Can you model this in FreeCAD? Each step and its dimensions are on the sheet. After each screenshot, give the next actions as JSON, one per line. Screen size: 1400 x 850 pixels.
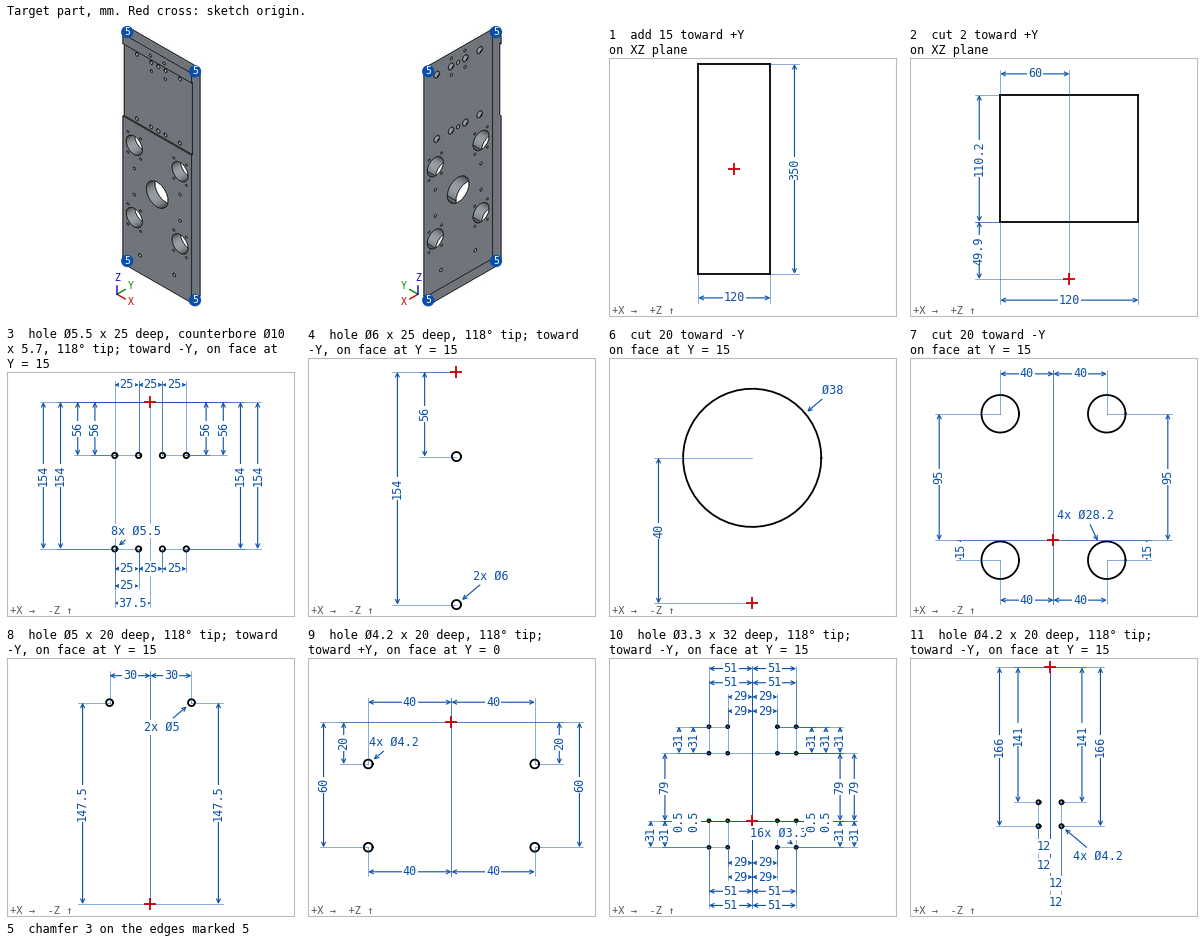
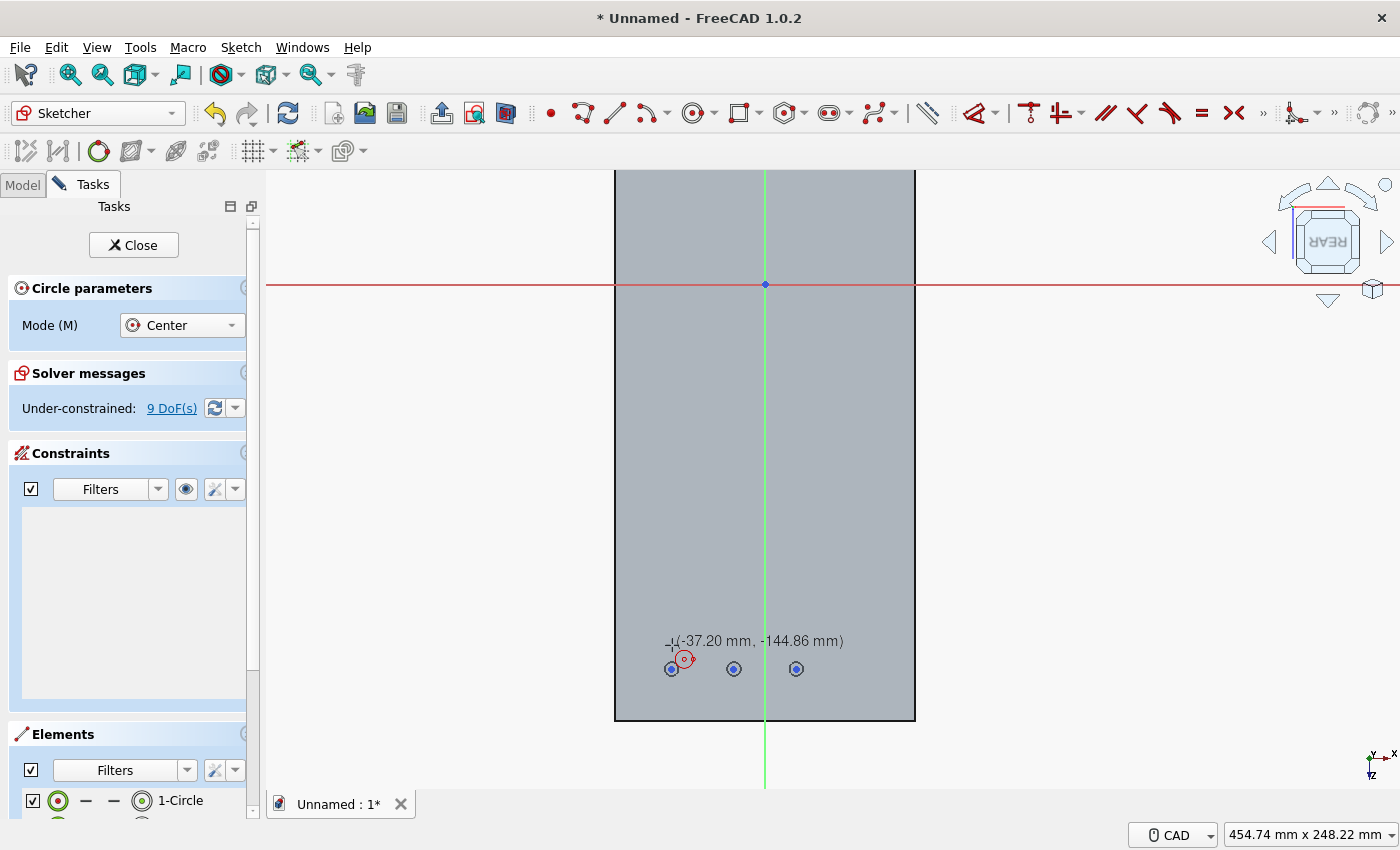
{"action": "scroll", "coordinate": [859, 669], "scroll_direction": "up", "scroll_amount": 6}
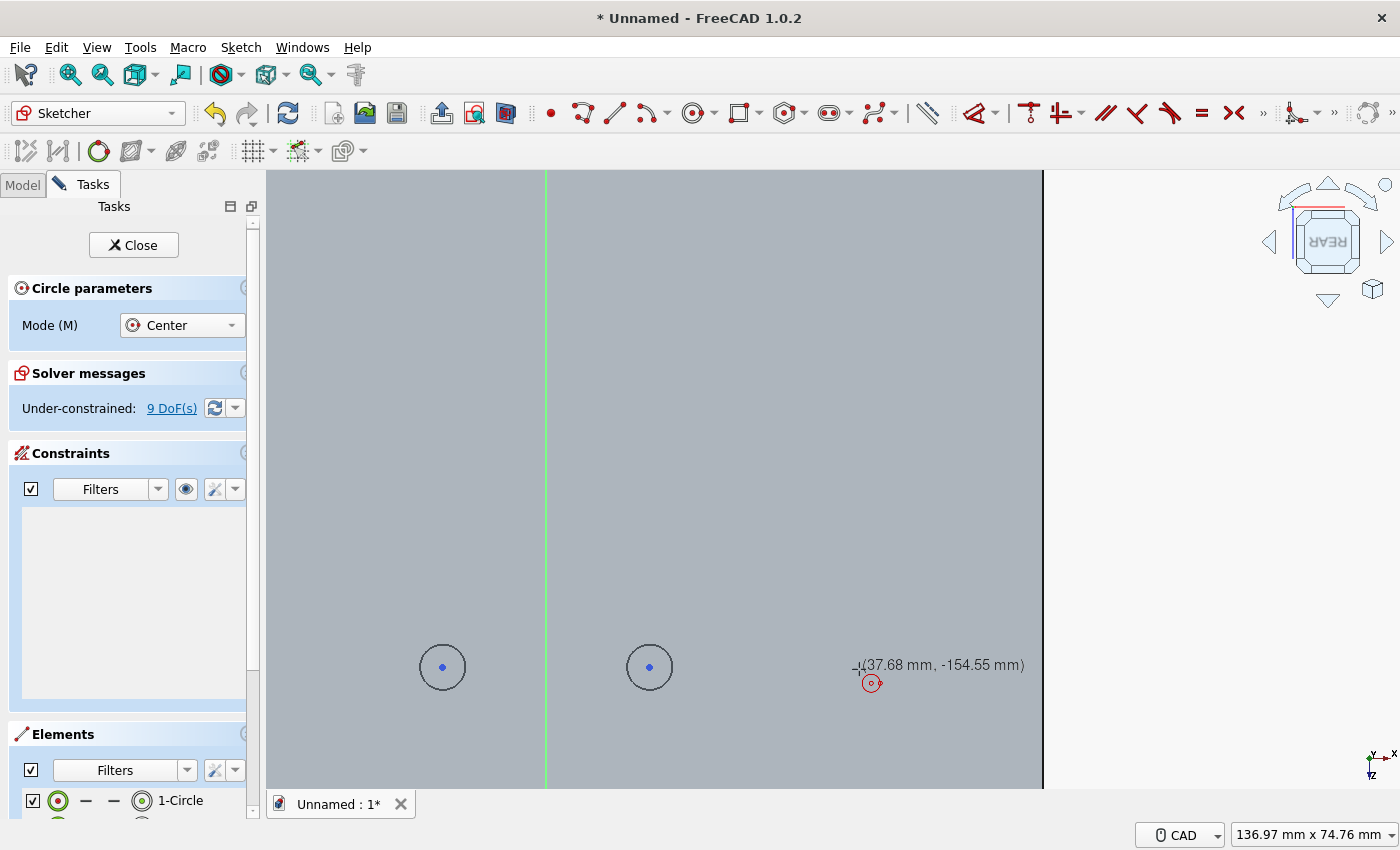
{"action": "left_click", "coordinate": [856, 666]}
{"action": "left_click", "coordinate": [872, 650]}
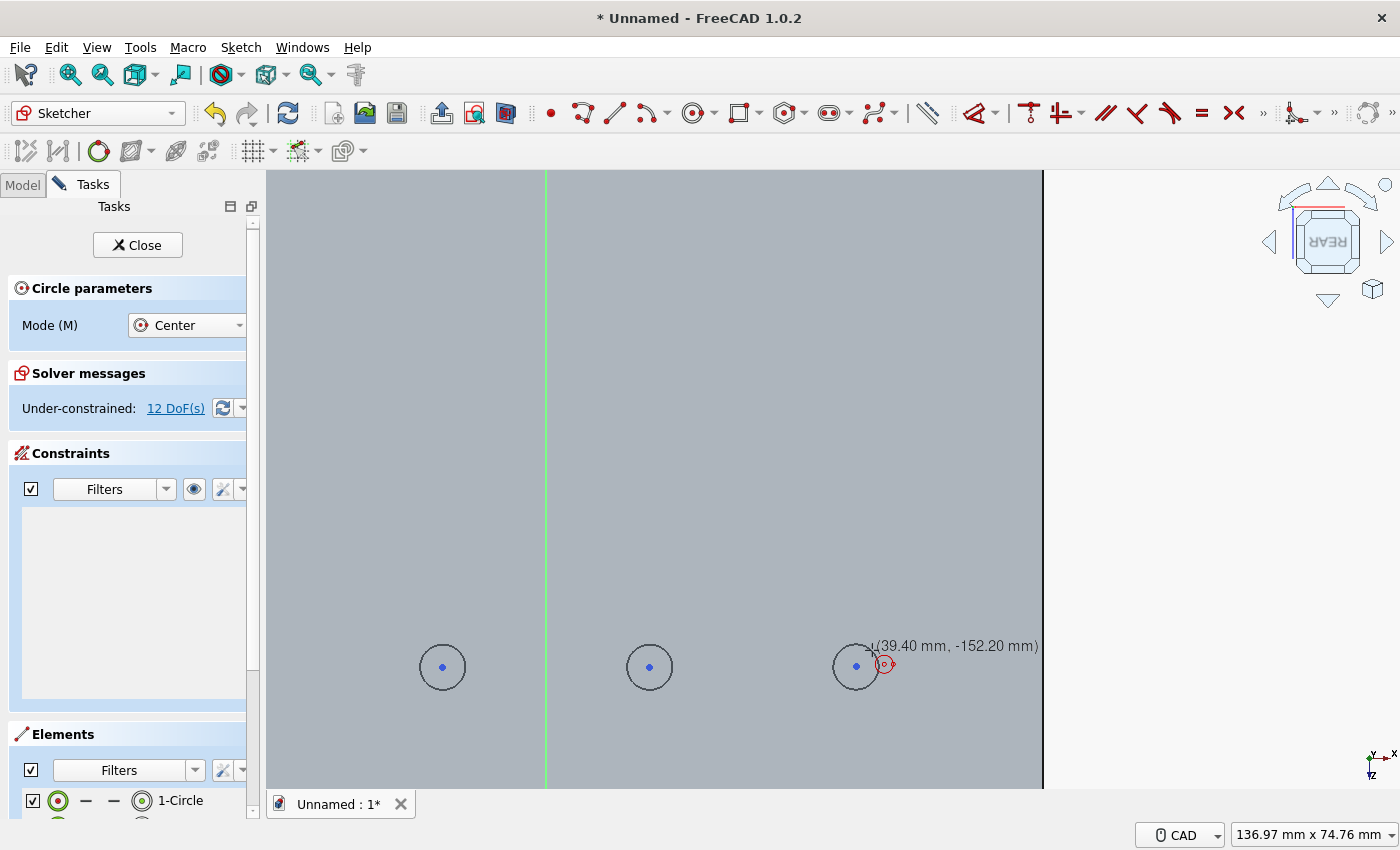
{"action": "scroll", "coordinate": [859, 669], "scroll_direction": "down", "scroll_amount": 6}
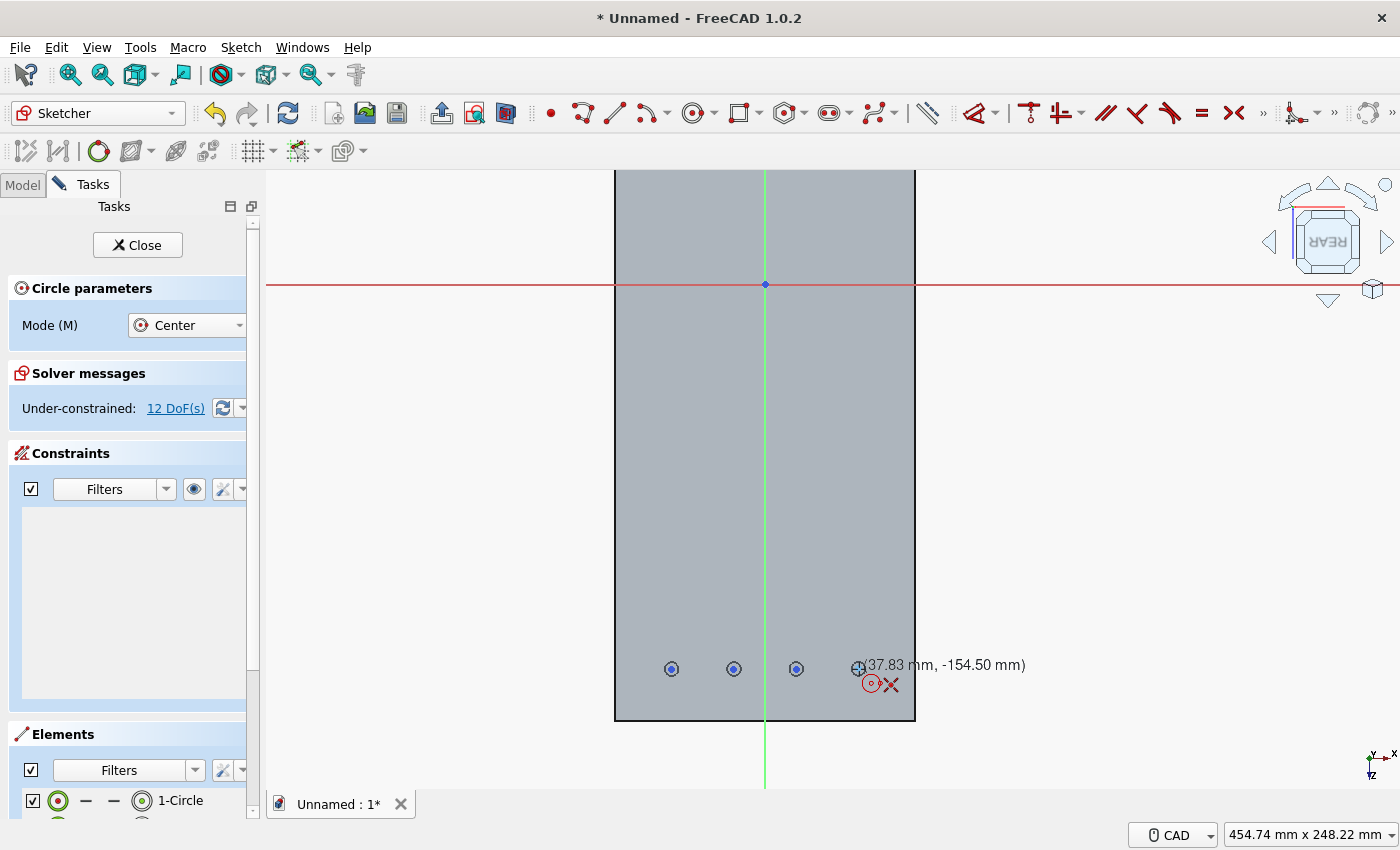
{"action": "scroll", "coordinate": [672, 424], "scroll_direction": "up", "scroll_amount": 6}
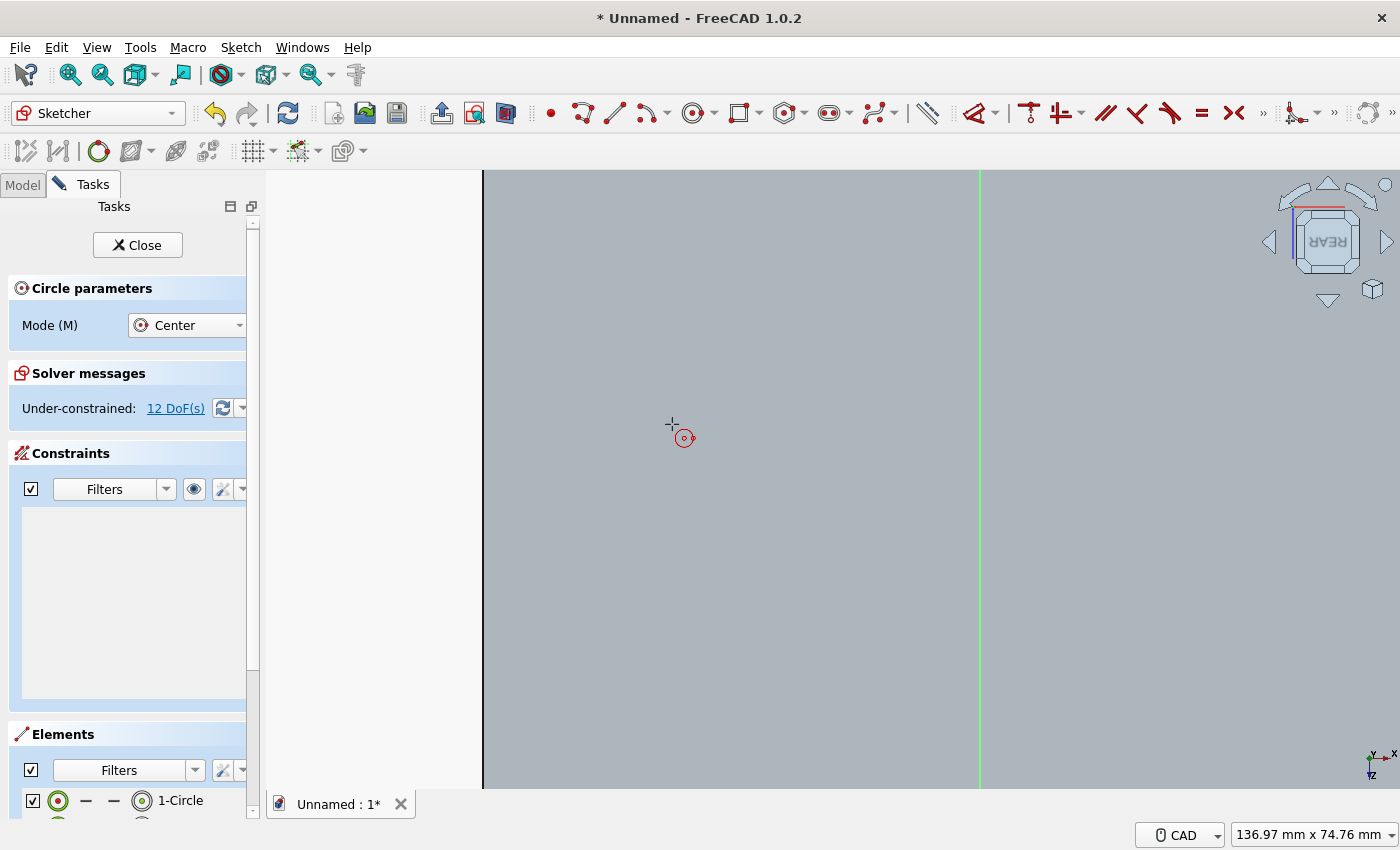
{"action": "left_click", "coordinate": [670, 424]}
{"action": "left_click", "coordinate": [686, 408]}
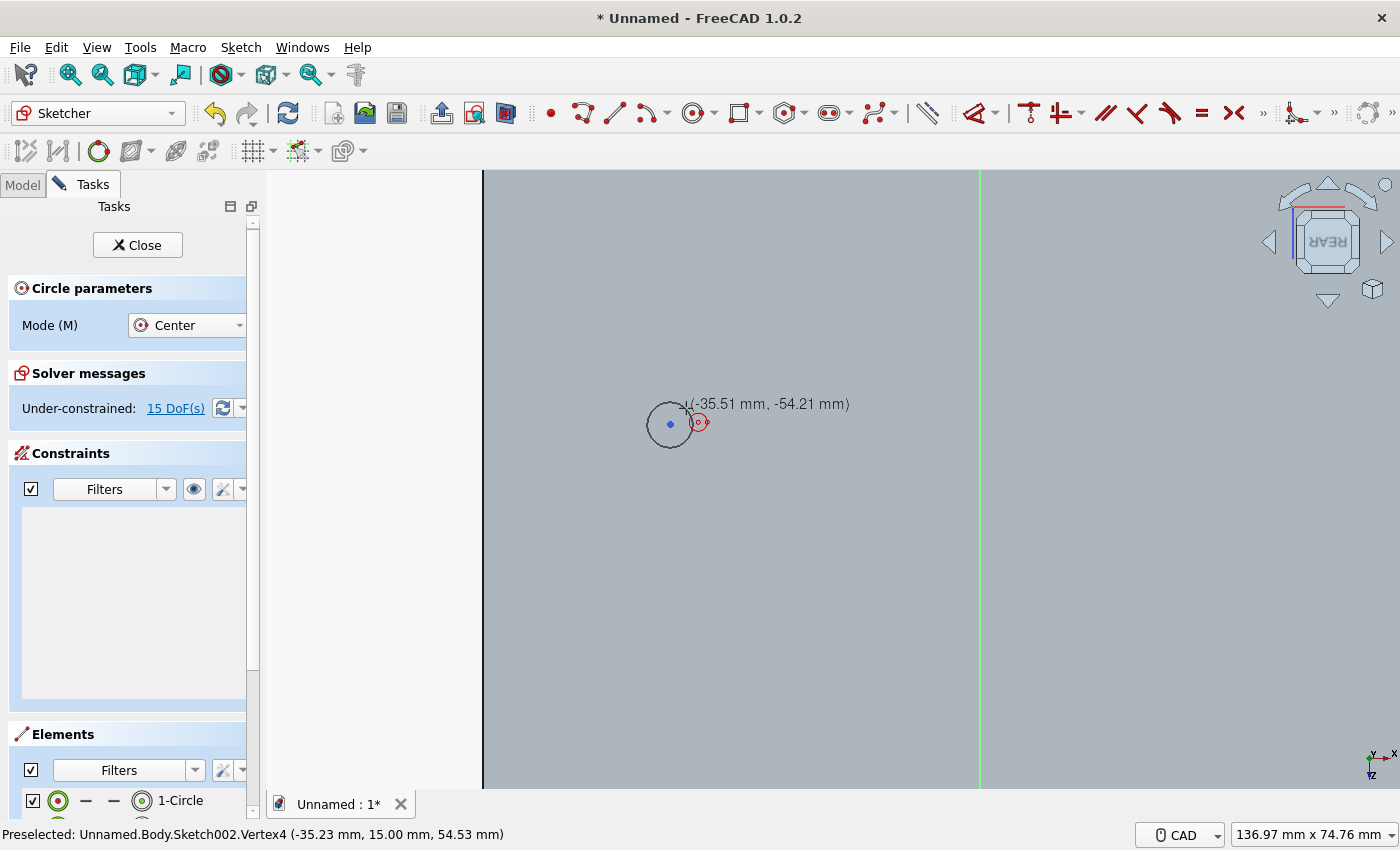
{"action": "left_click", "coordinate": [877, 424]}
{"action": "left_click", "coordinate": [893, 408]}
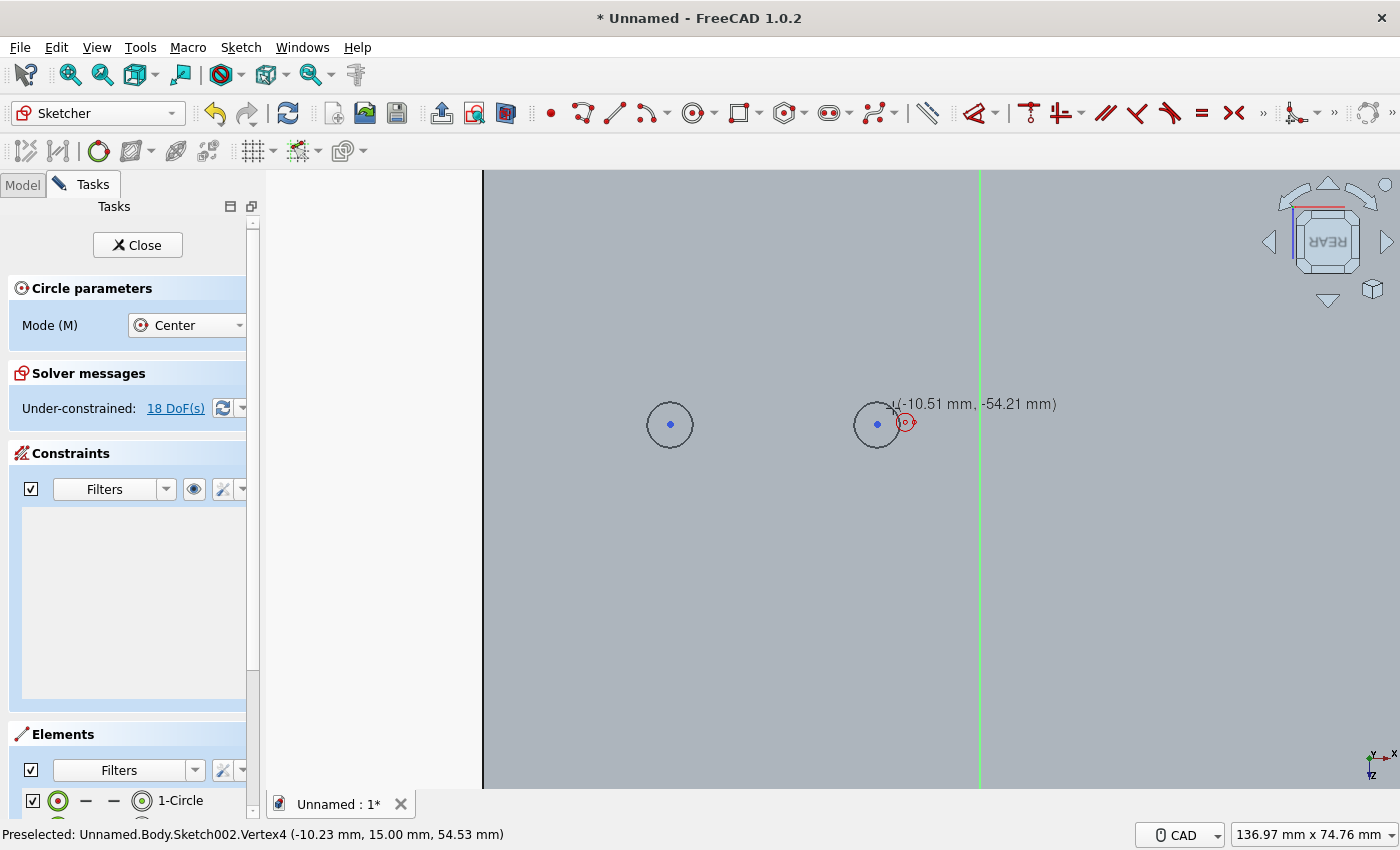
{"action": "left_click", "coordinate": [1084, 424]}
{"action": "left_click", "coordinate": [1100, 408]}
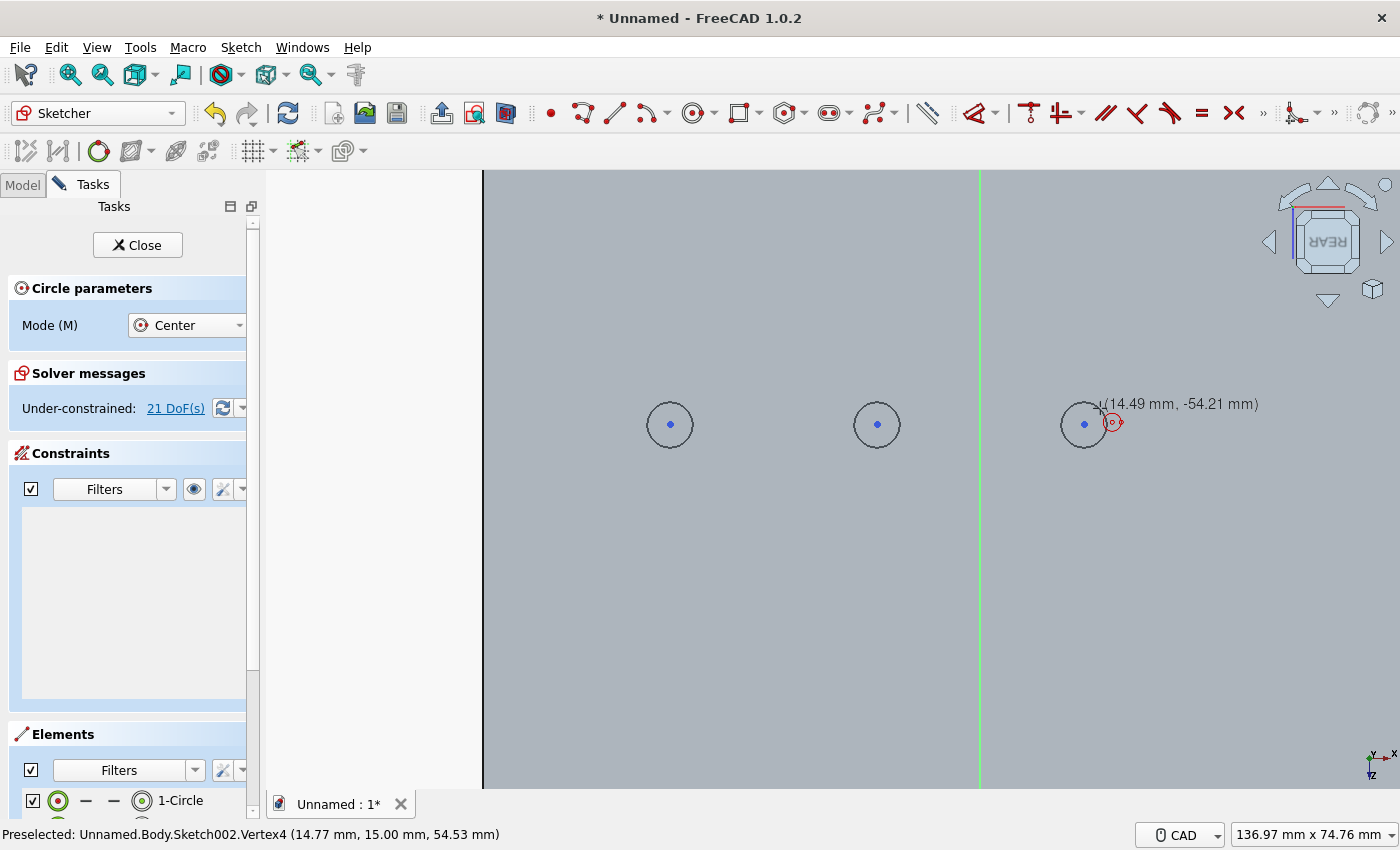
{"action": "scroll", "coordinate": [672, 424], "scroll_direction": "down", "scroll_amount": 6}